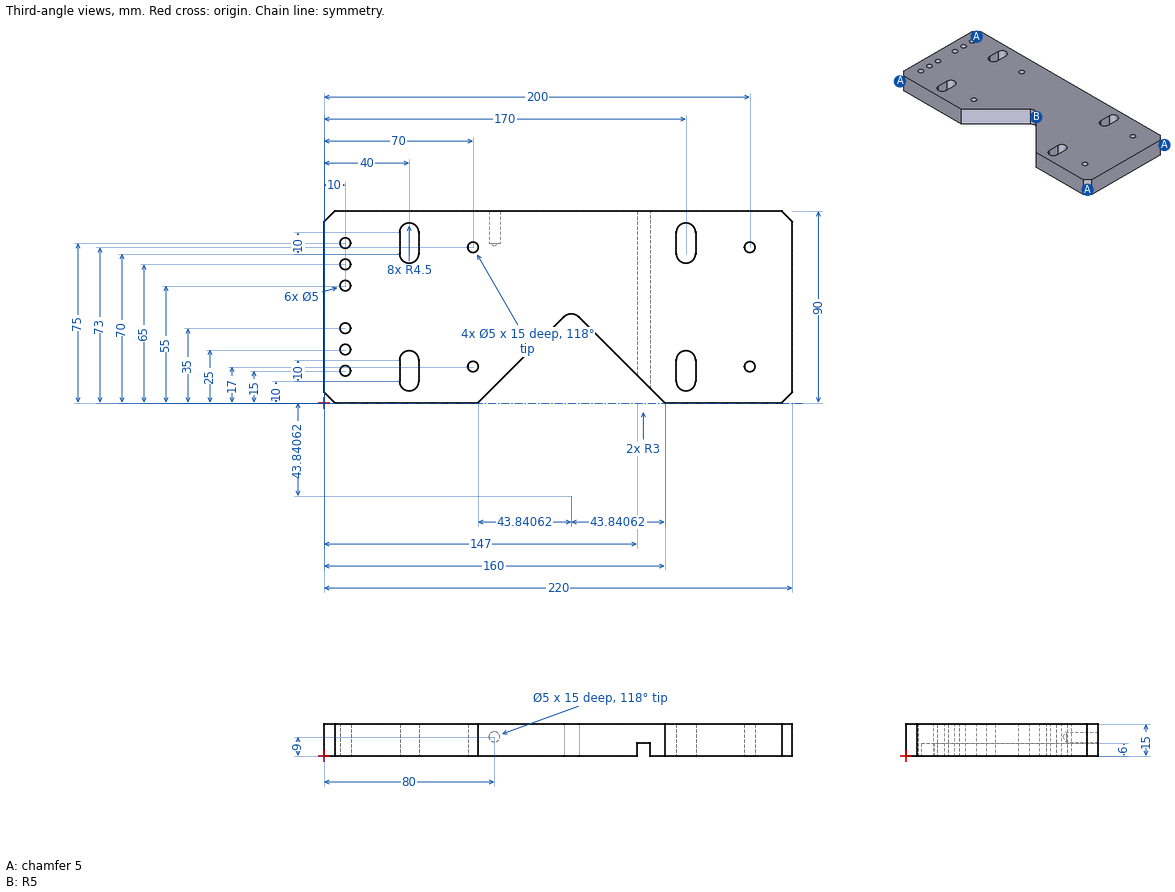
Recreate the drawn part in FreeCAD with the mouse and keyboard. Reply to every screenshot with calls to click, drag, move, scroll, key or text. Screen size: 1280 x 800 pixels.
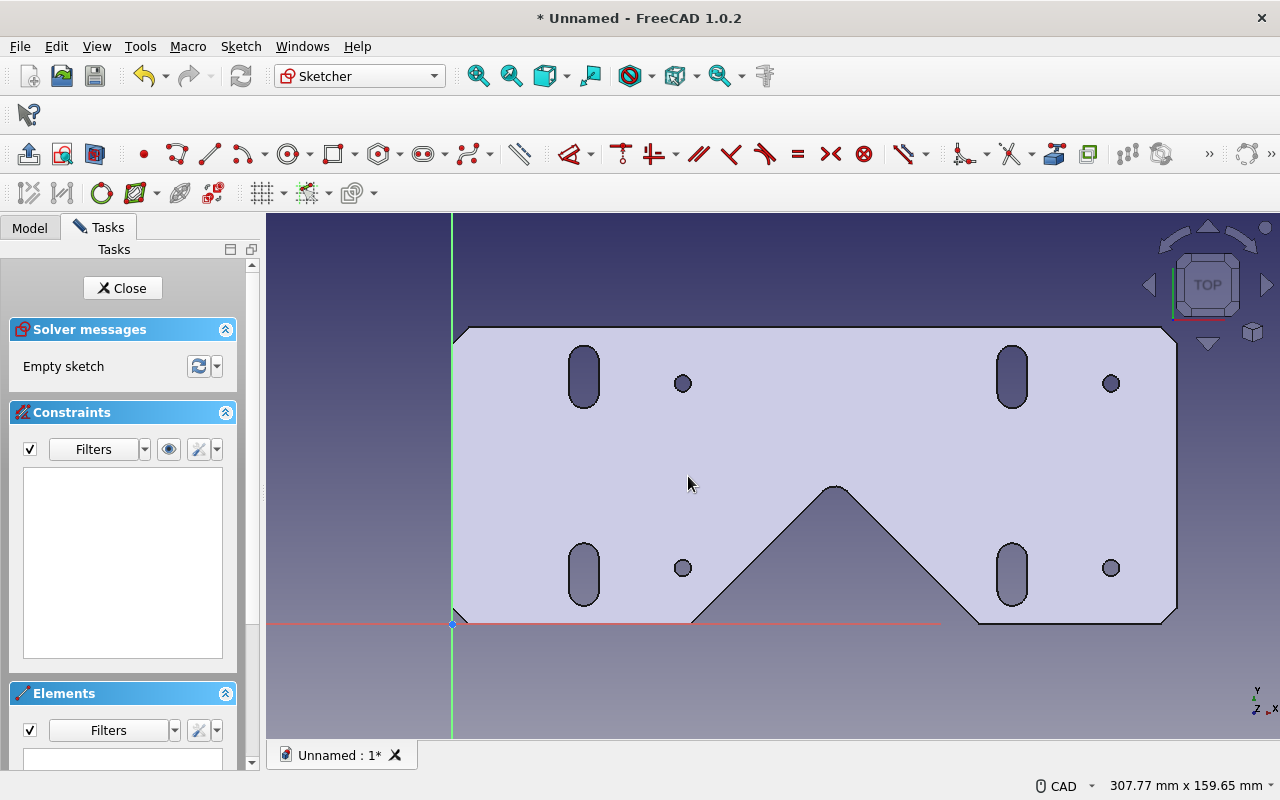
key(g)
key(s)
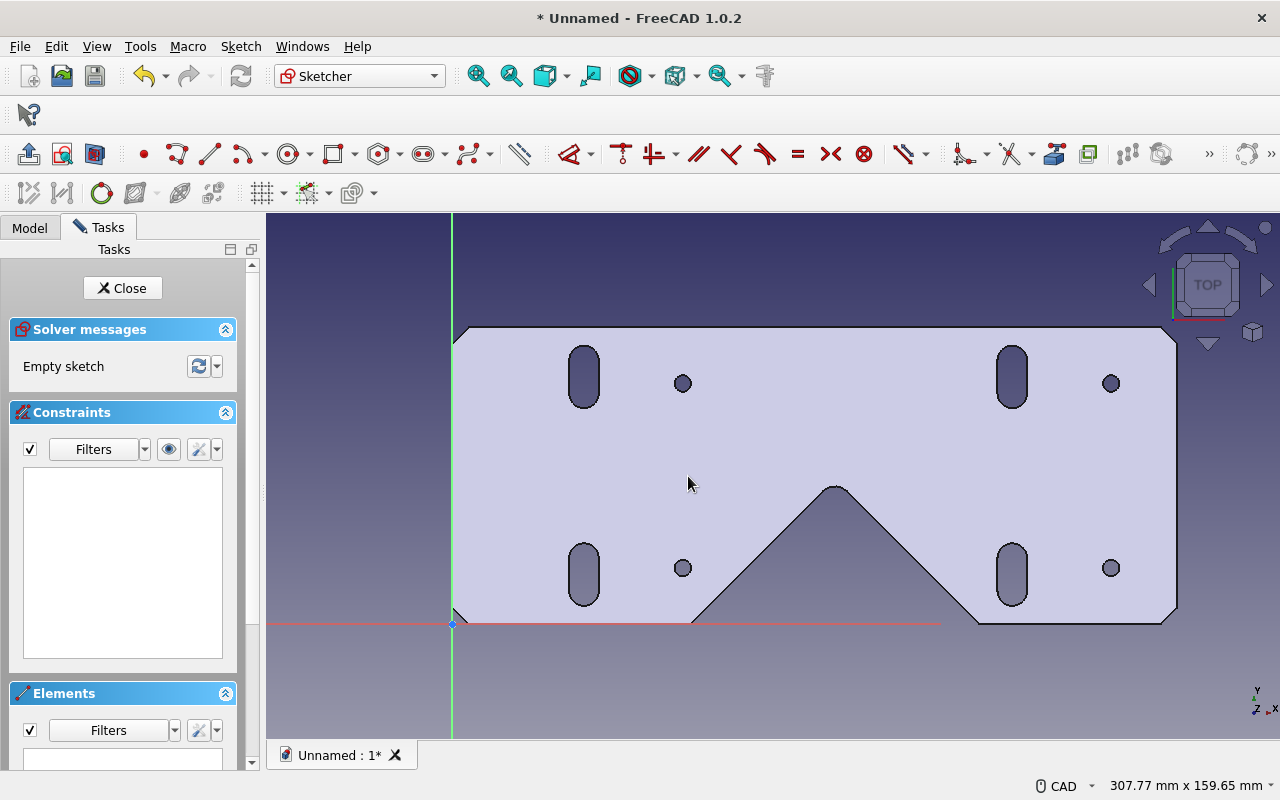
scroll(946, 624, up, 5)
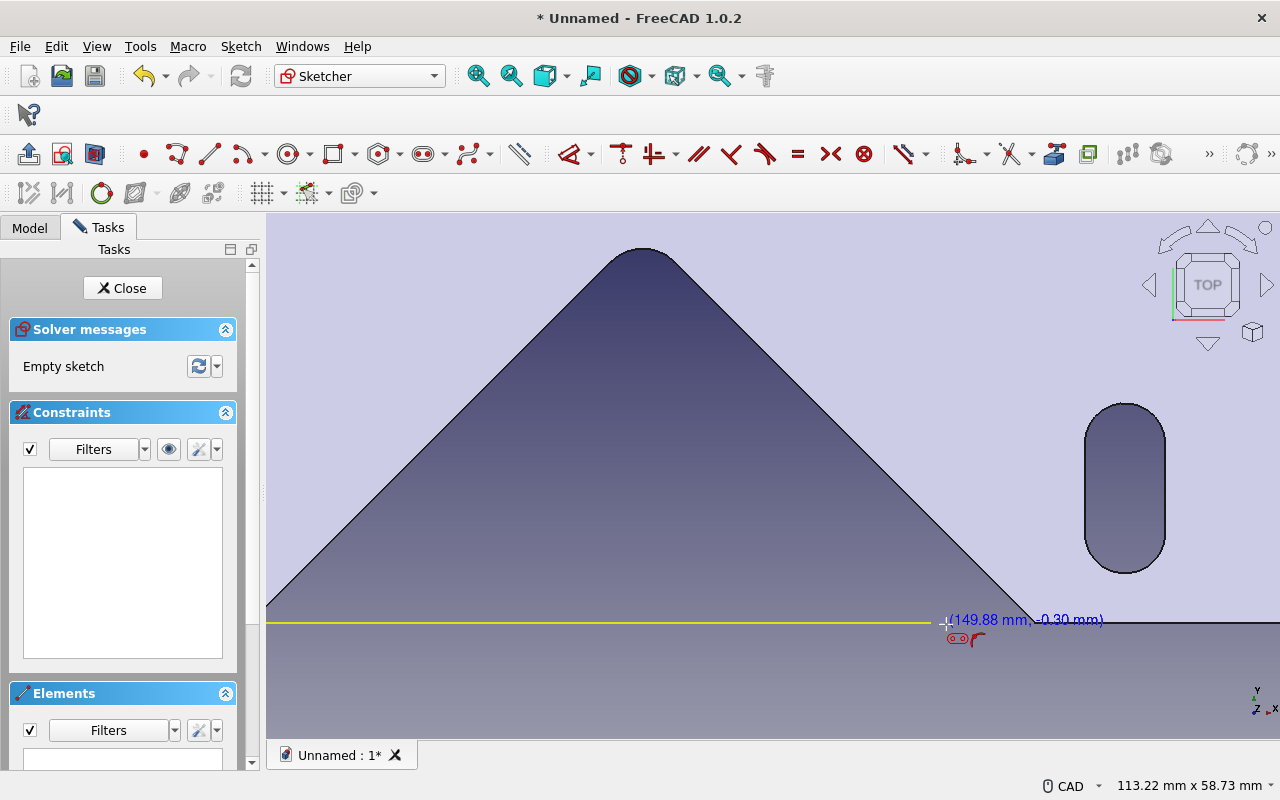
click(946, 623)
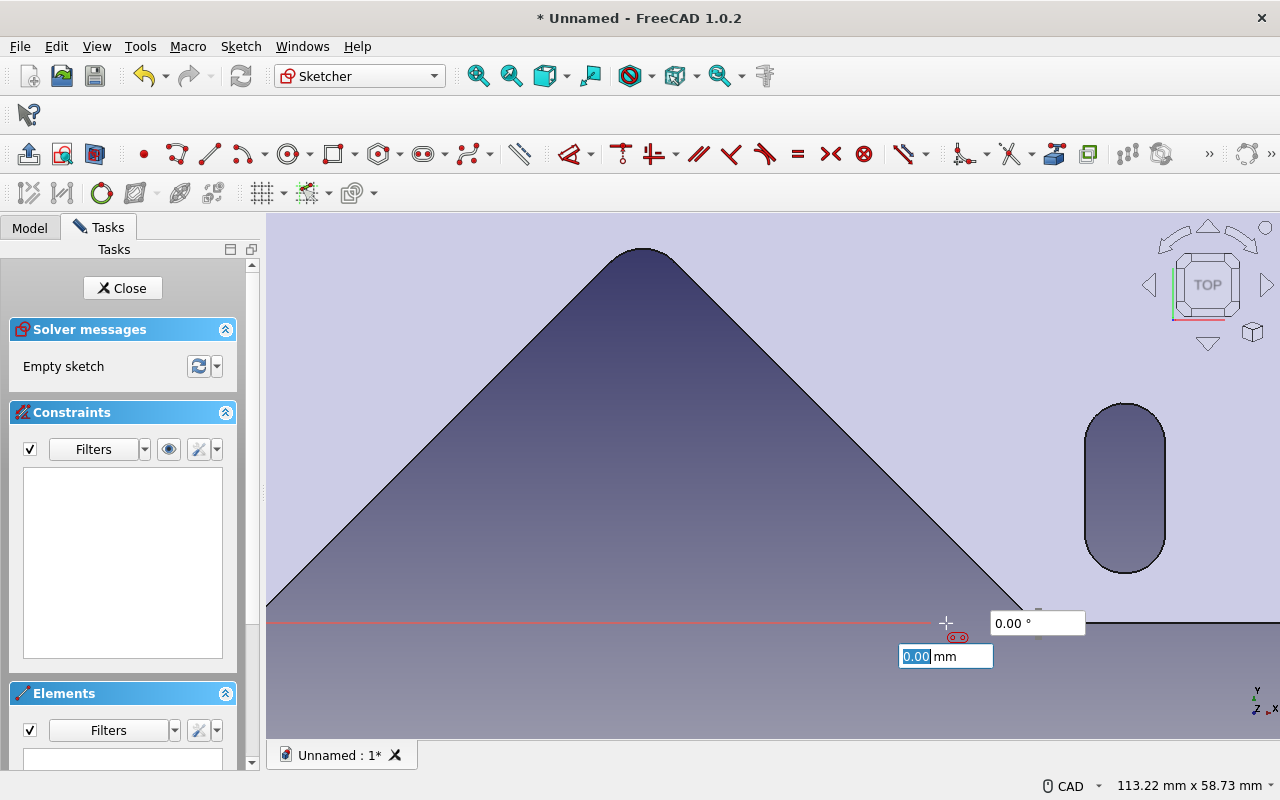
scroll(947, 625, down, 5)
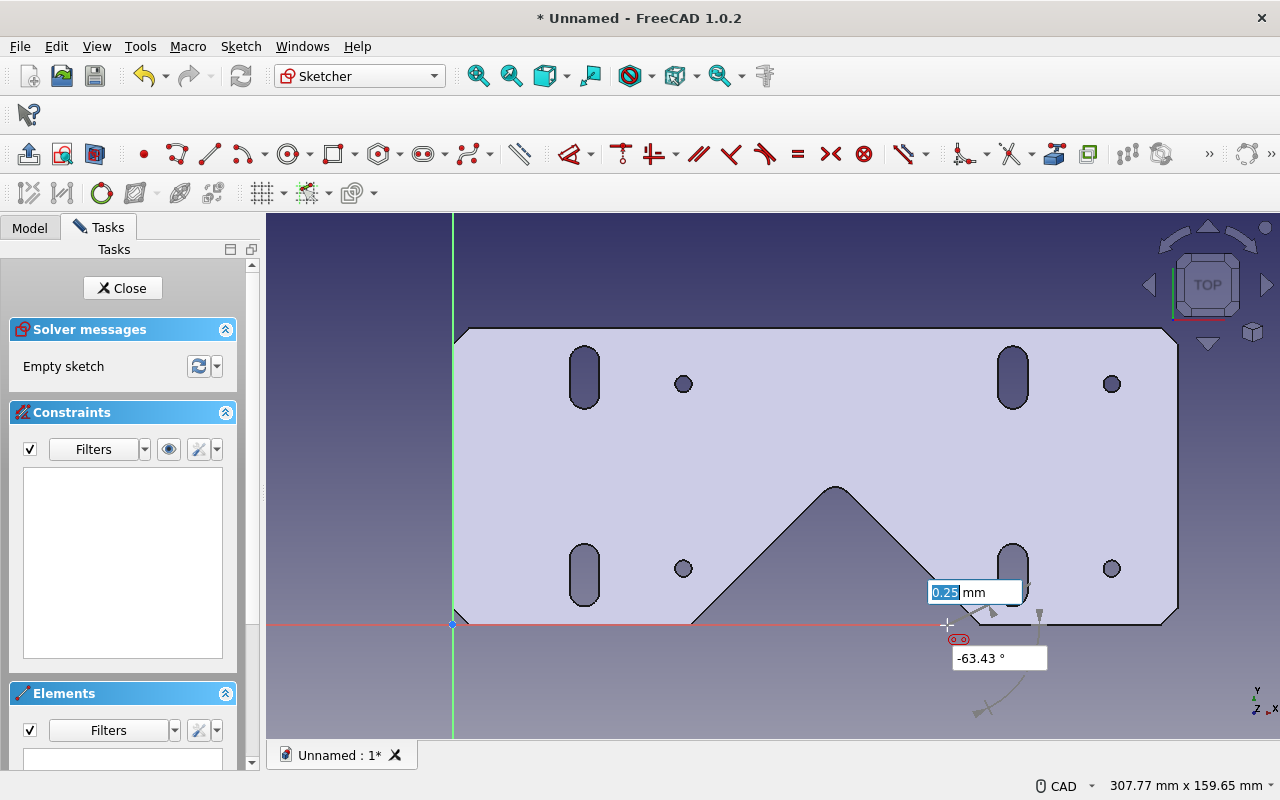
click(947, 328)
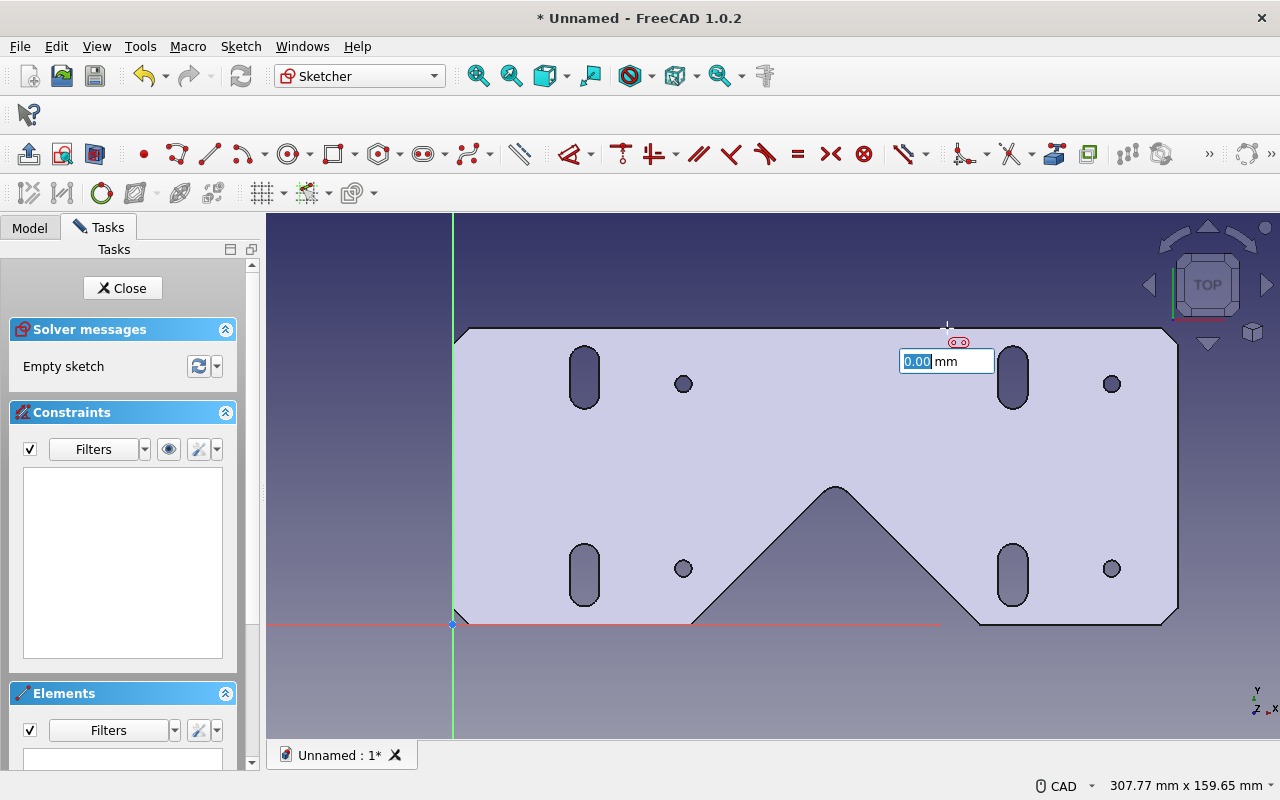
scroll(957, 476, up, 3)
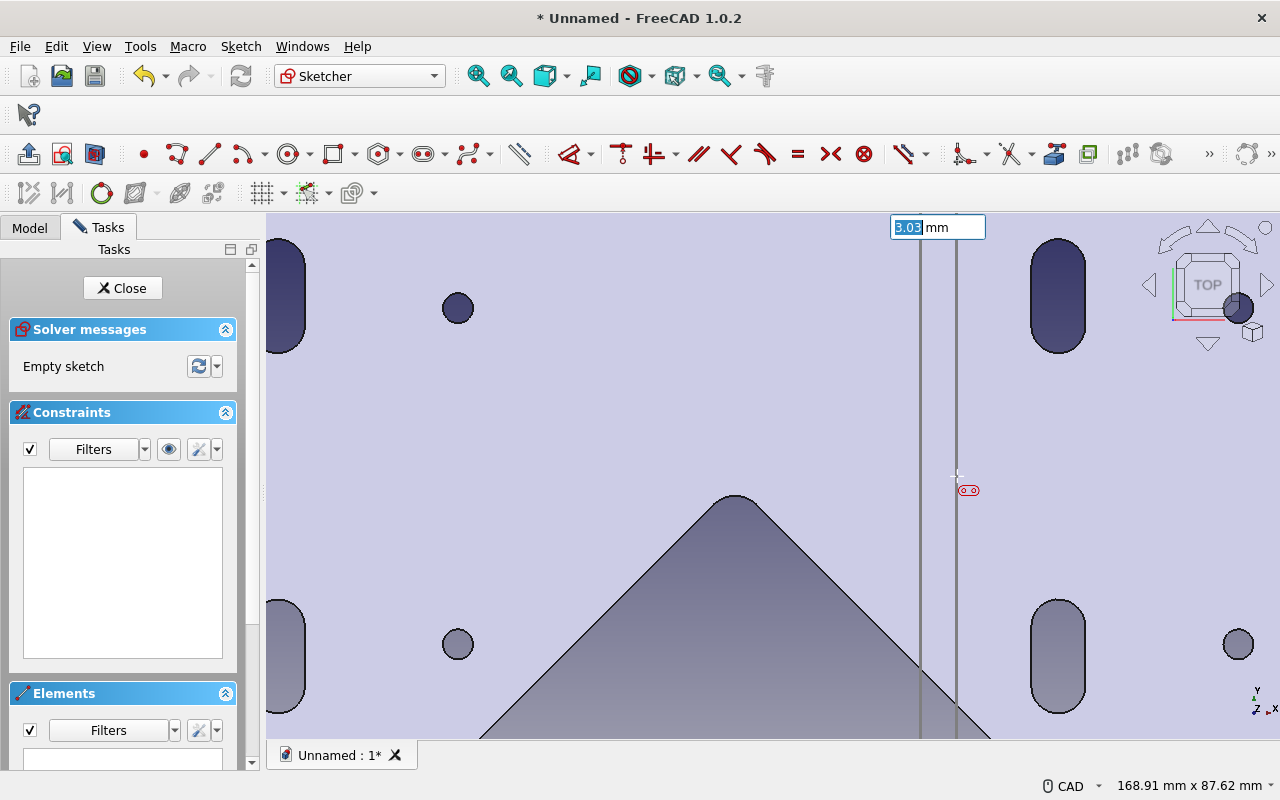
click(956, 476)
key(Escape)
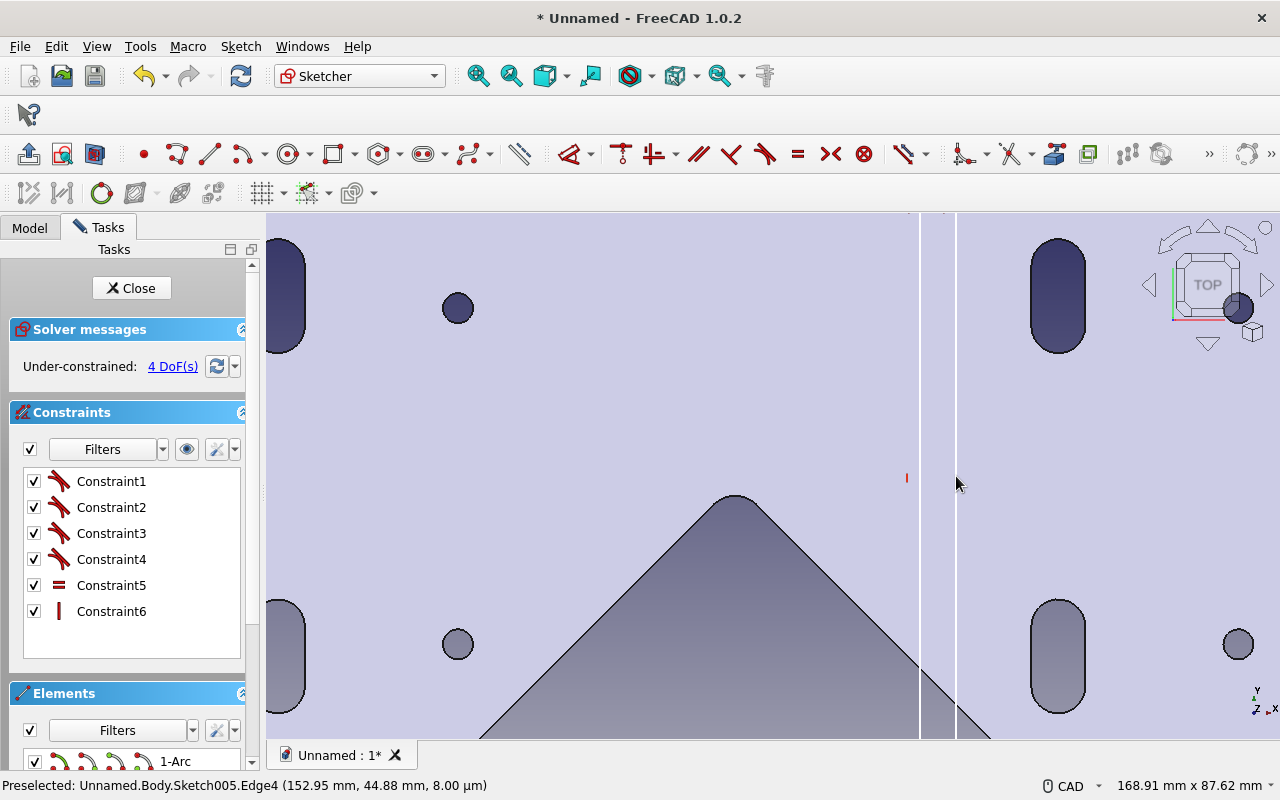
scroll(957, 476, down, 3)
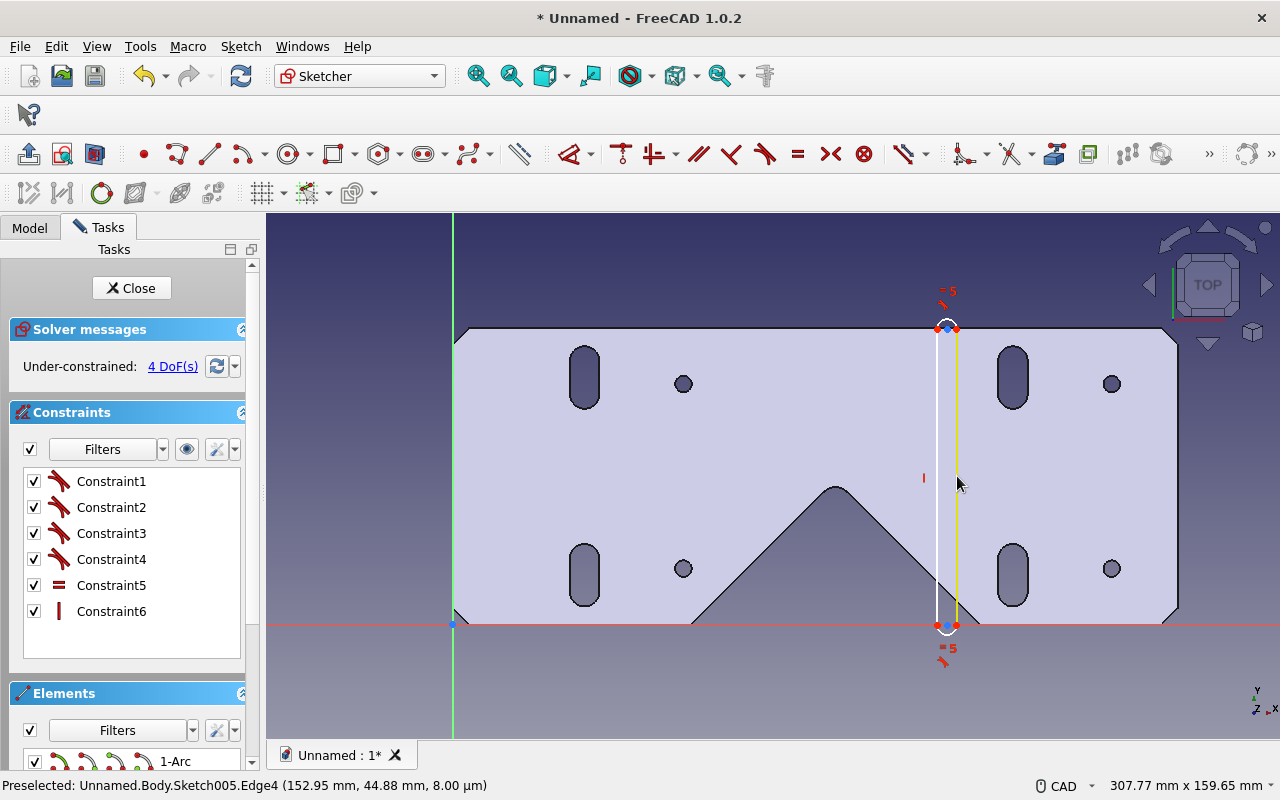
scroll(947, 625, up, 2)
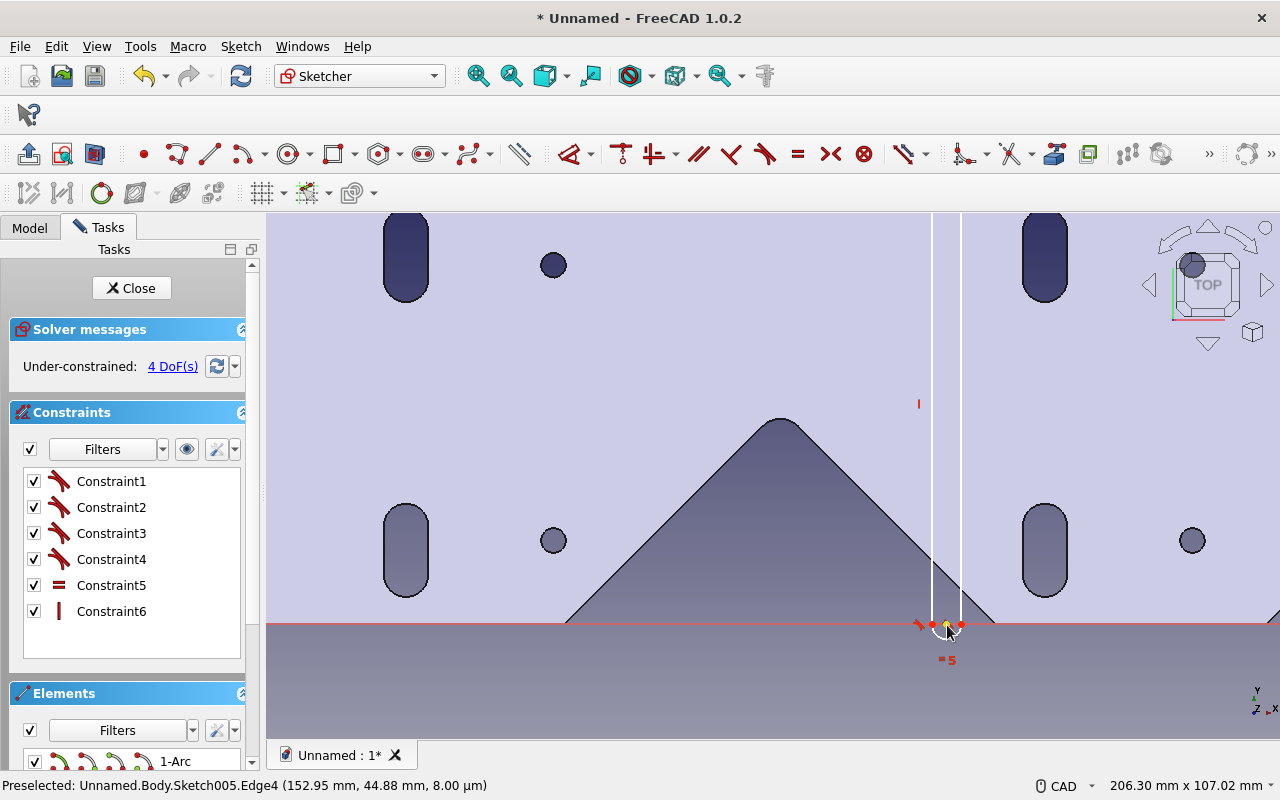
click(947, 625)